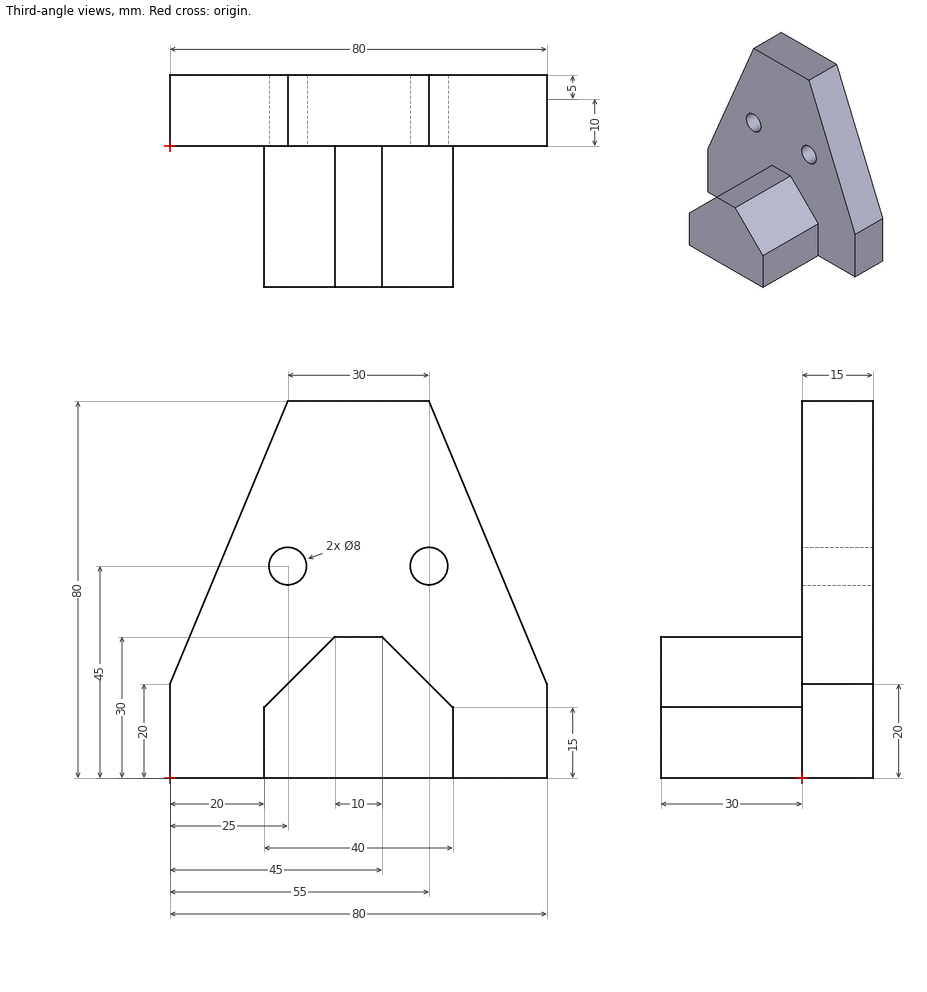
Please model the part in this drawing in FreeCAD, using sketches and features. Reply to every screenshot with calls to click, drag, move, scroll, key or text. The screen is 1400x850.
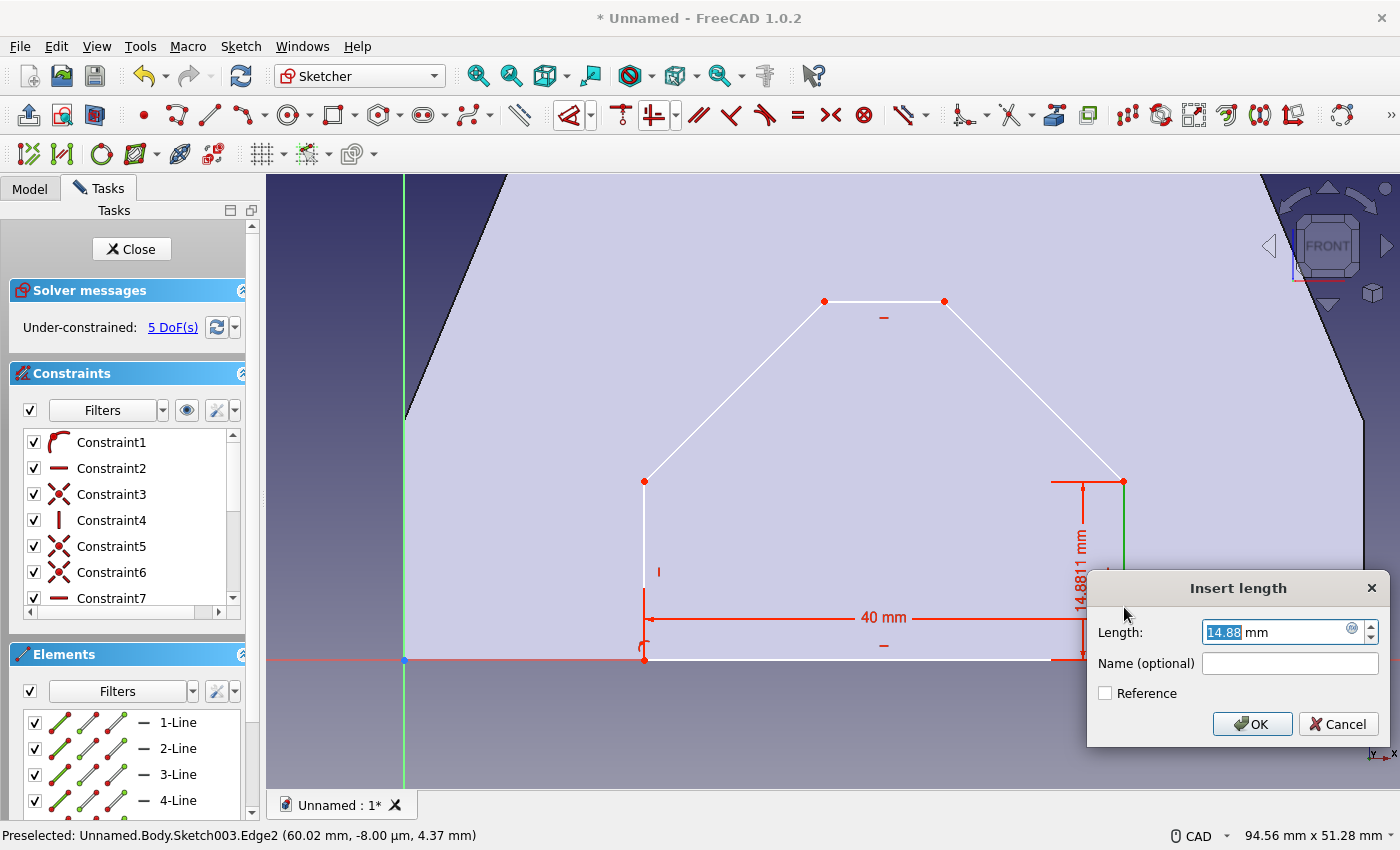
text(15)
key(Return)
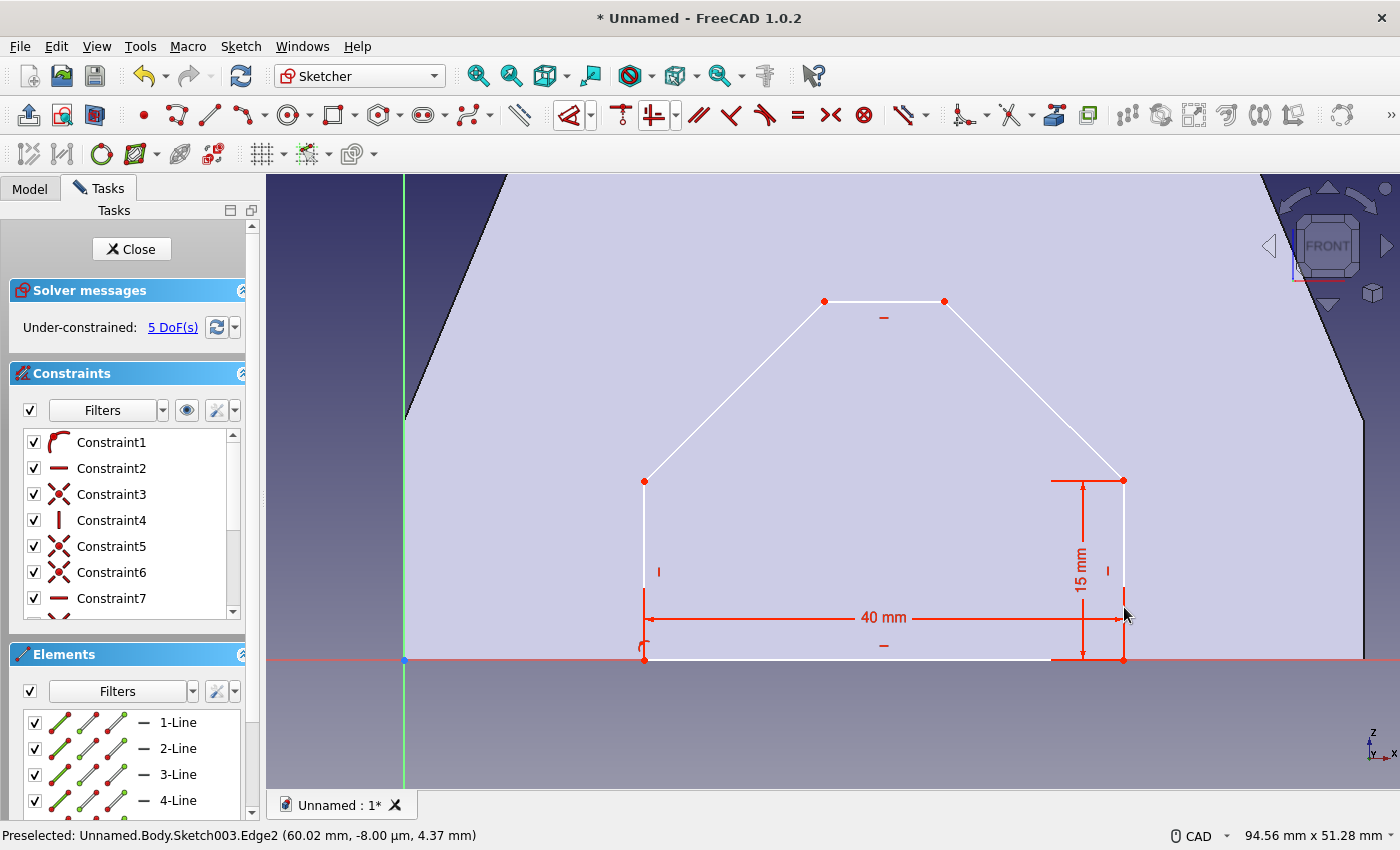
click(908, 302)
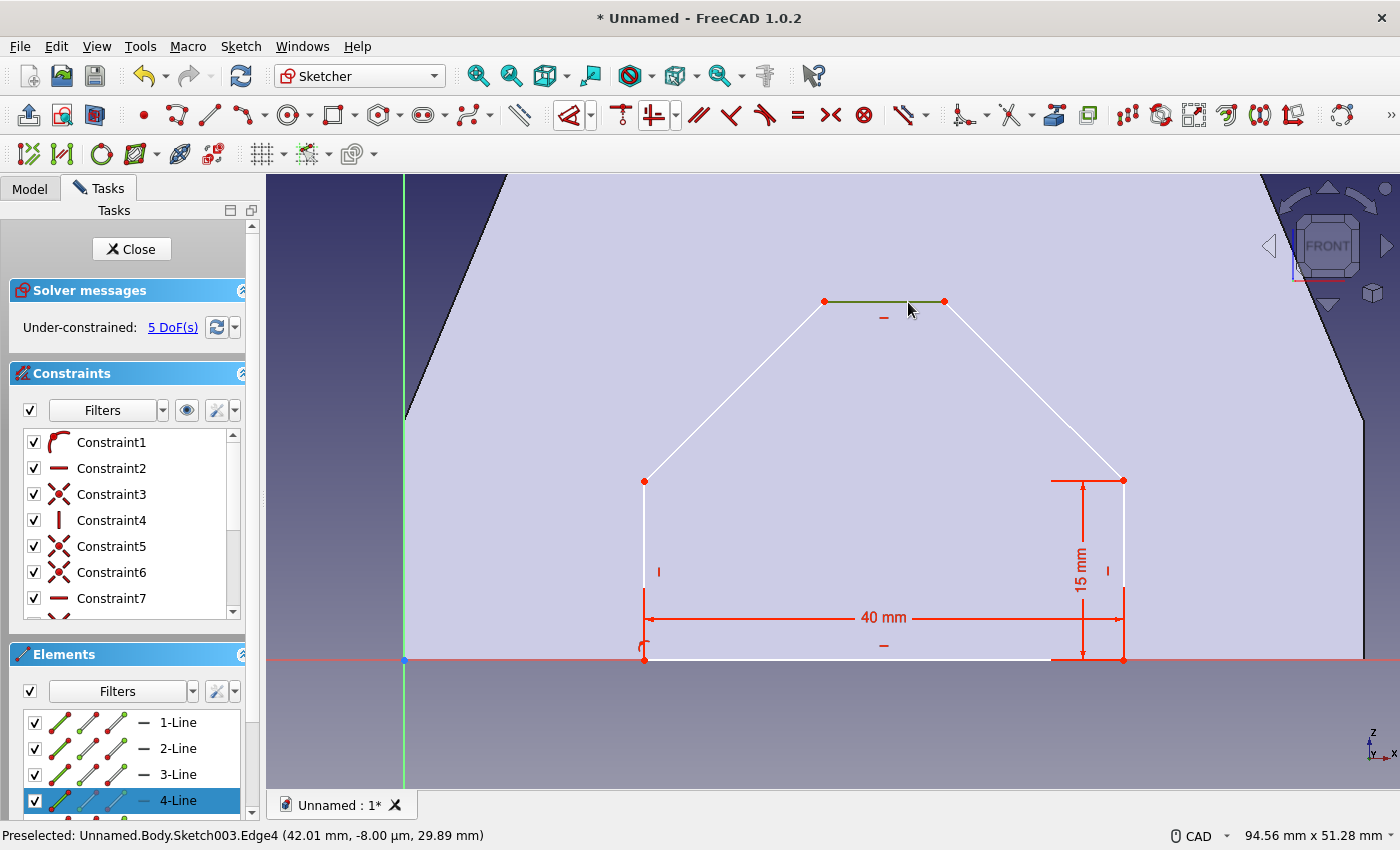
click(590, 116)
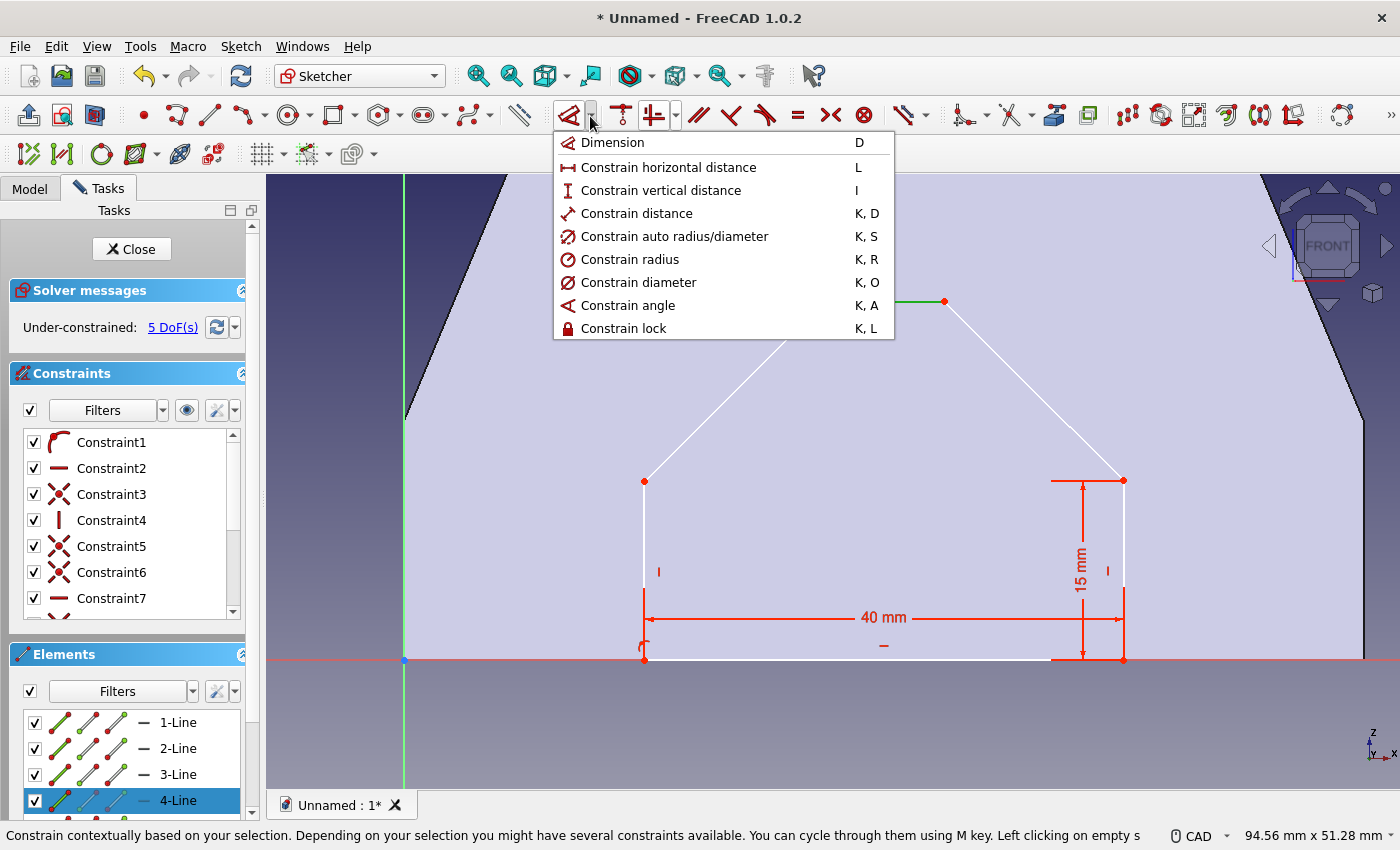
click(724, 168)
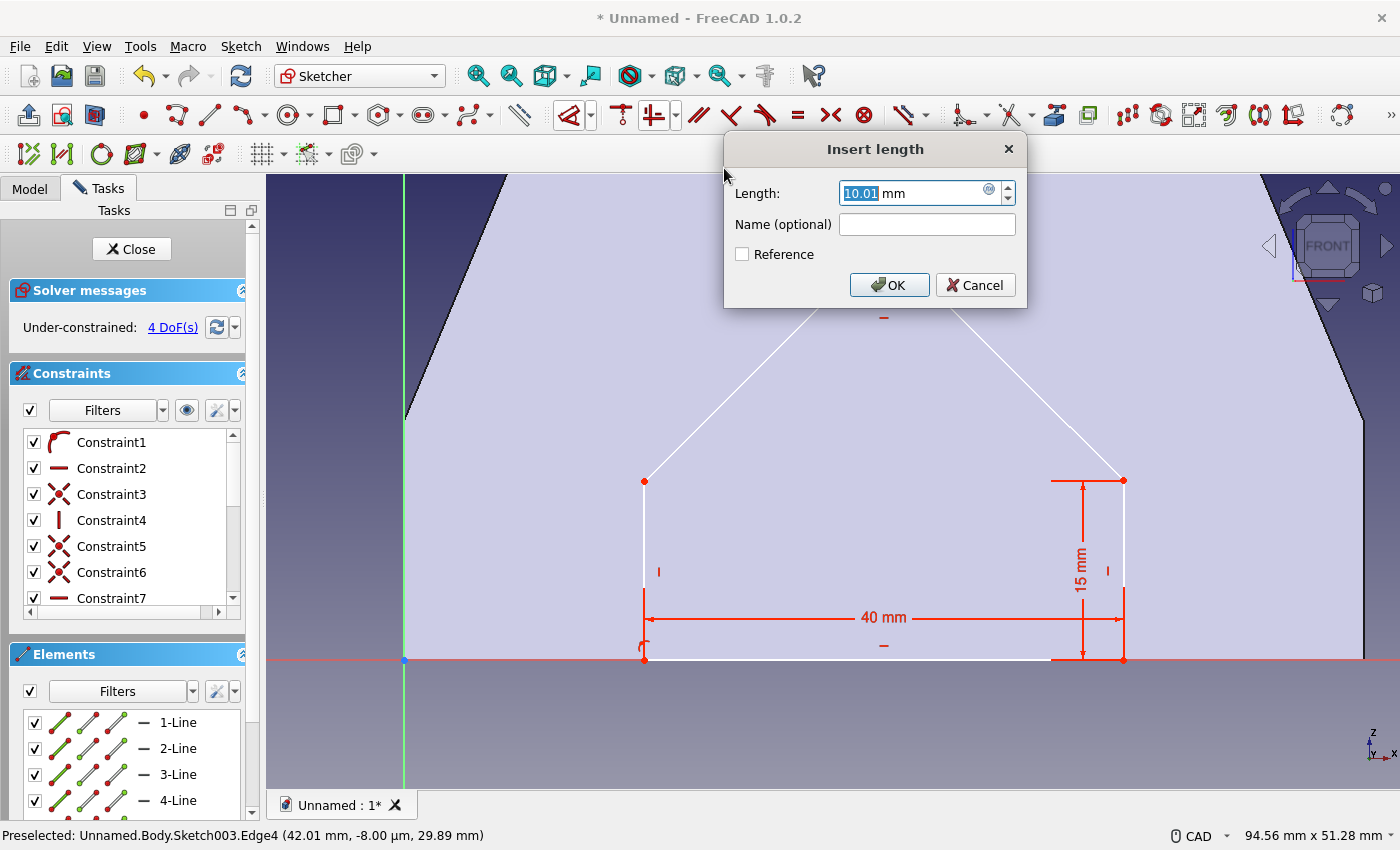
text(10)
key(Return)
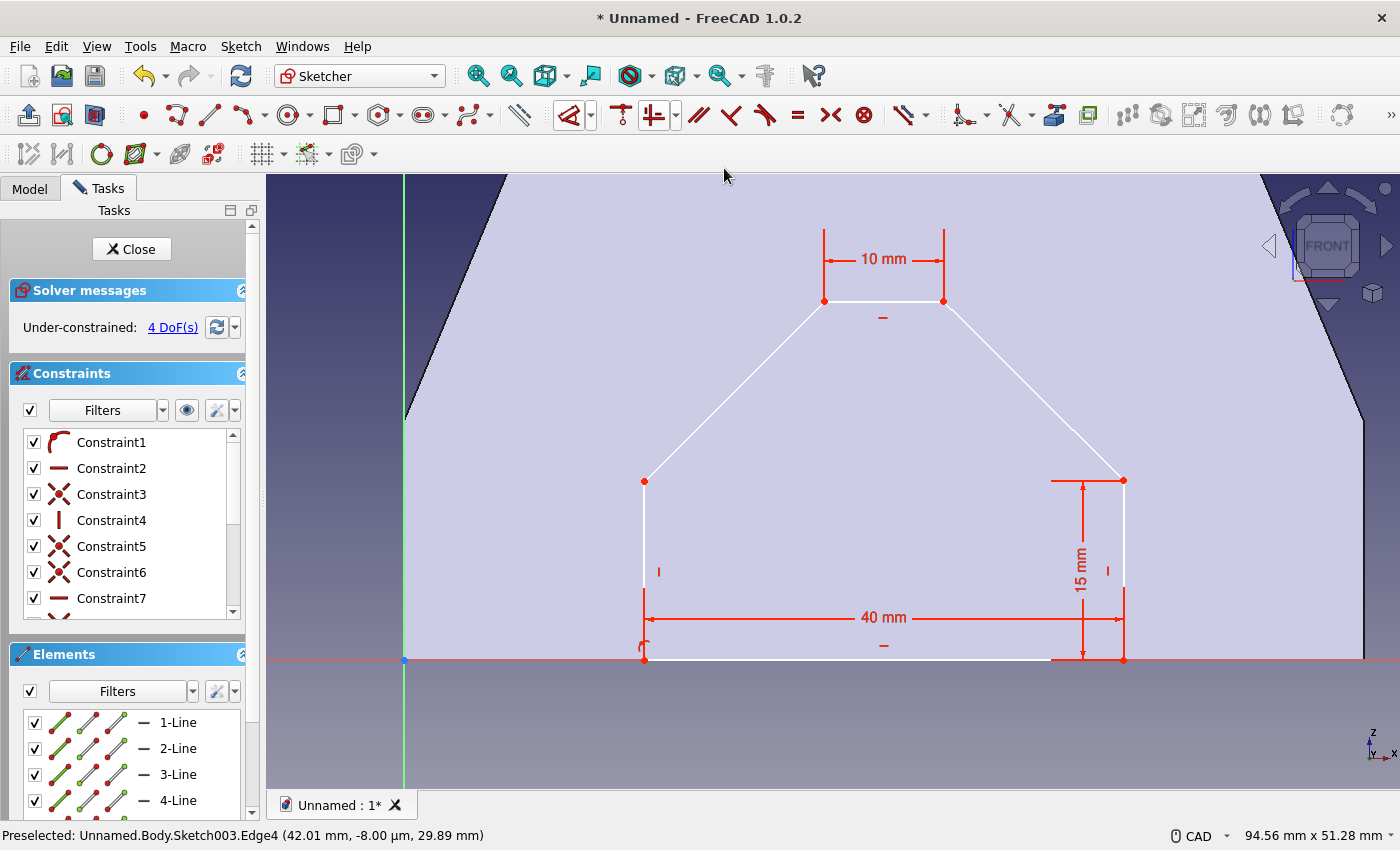
click(644, 536)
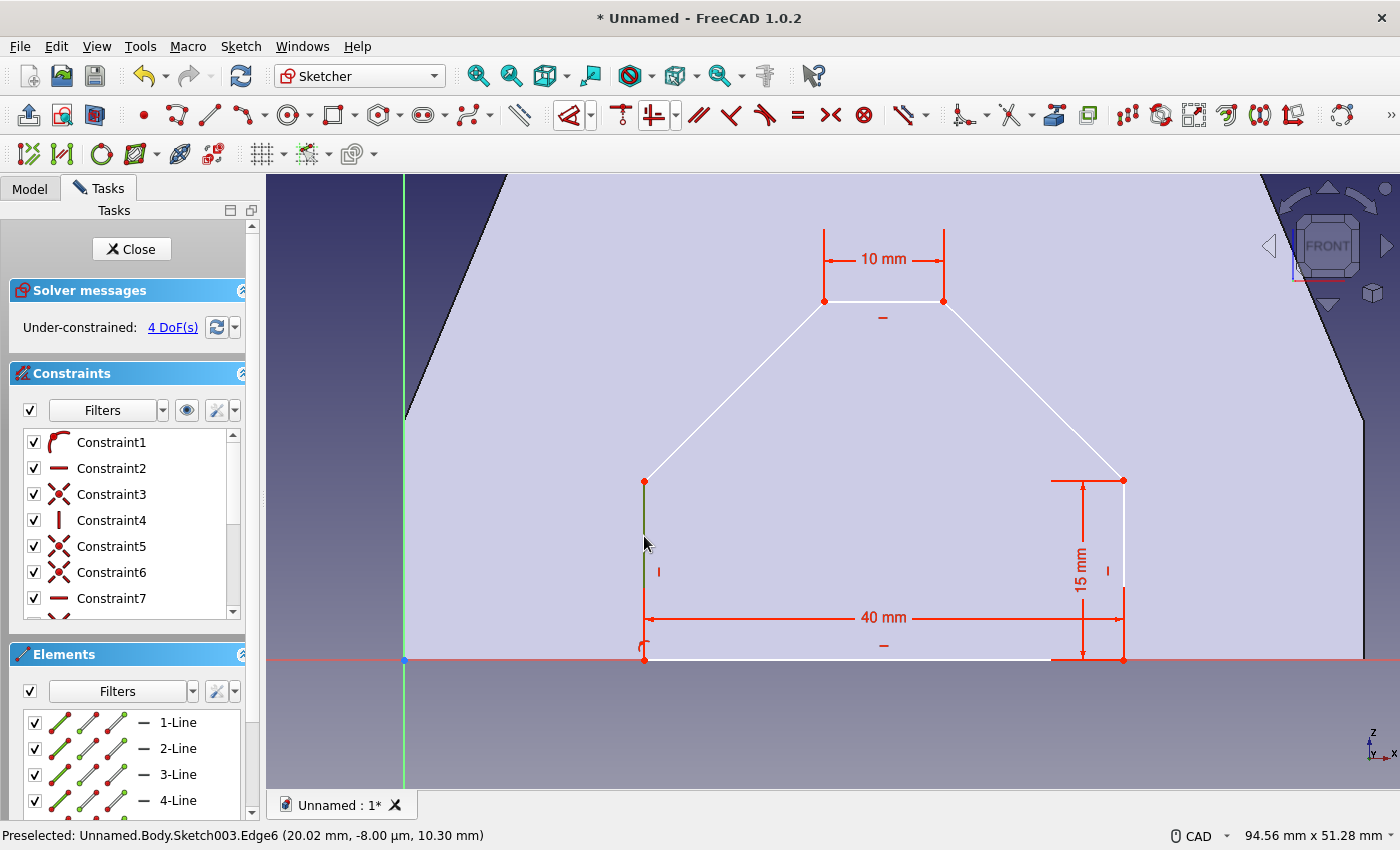
key(i)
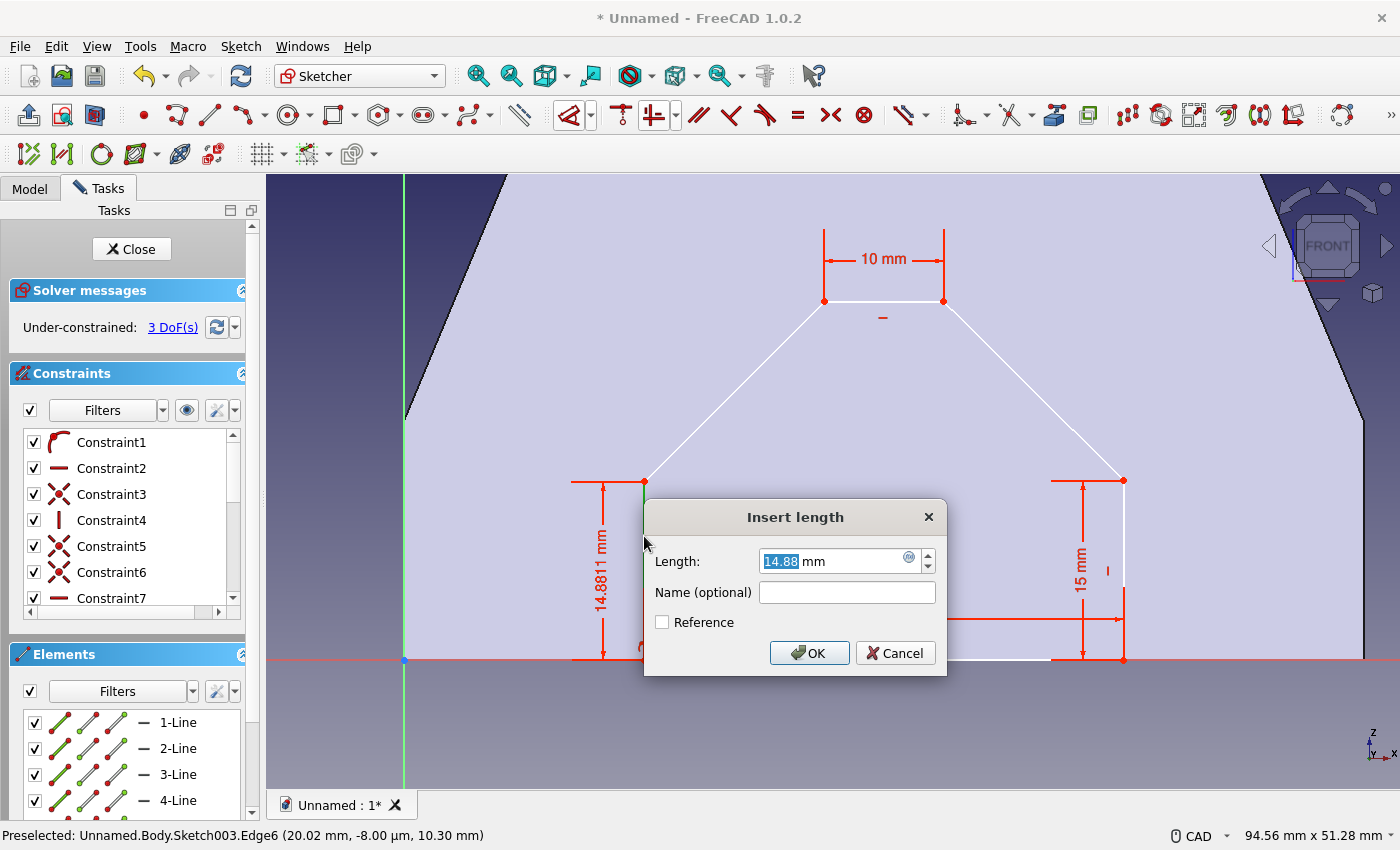
text(15)
key(Return)